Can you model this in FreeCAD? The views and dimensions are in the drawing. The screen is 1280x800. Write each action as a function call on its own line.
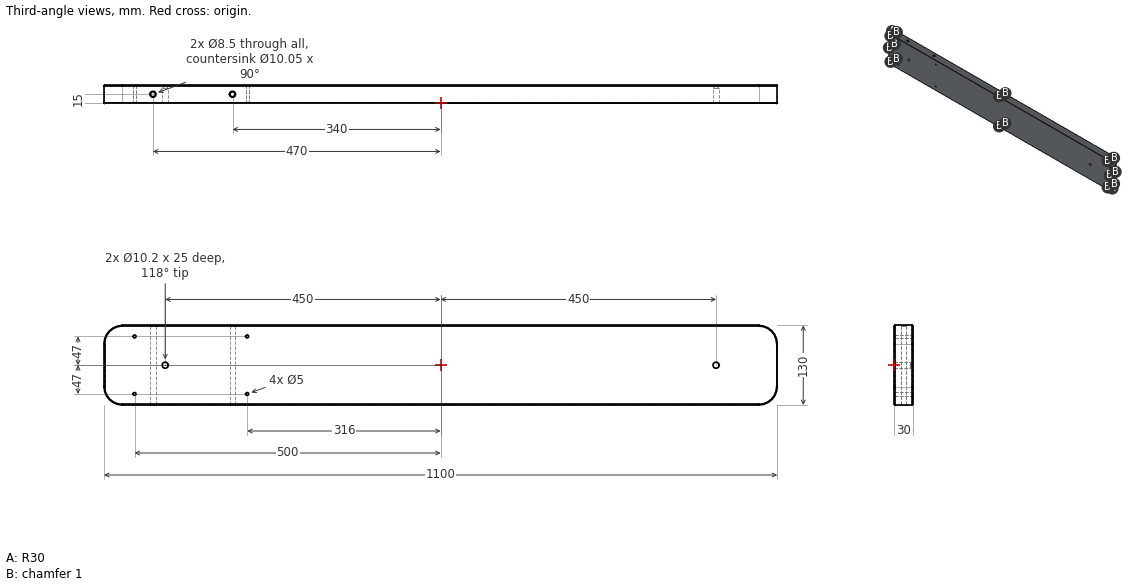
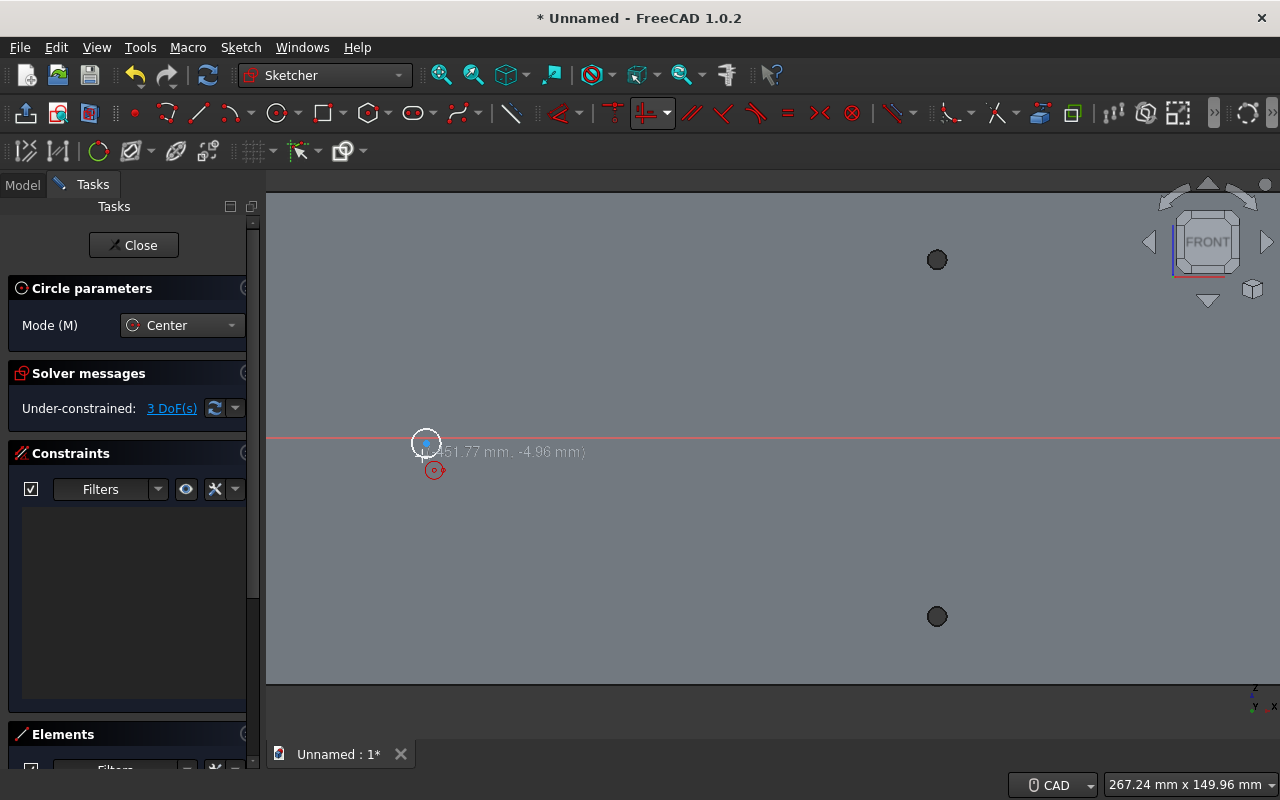
scroll(421, 458, down, 9)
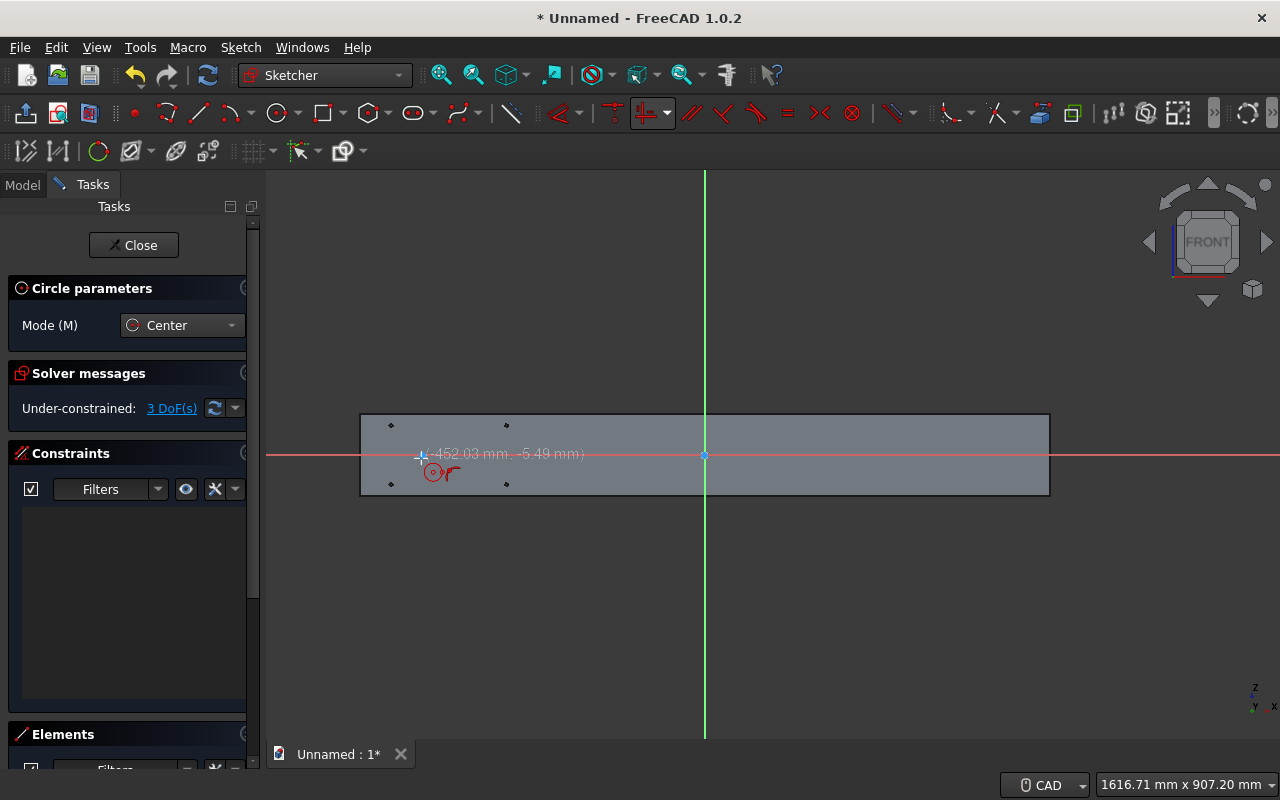
scroll(987, 455, up, 10)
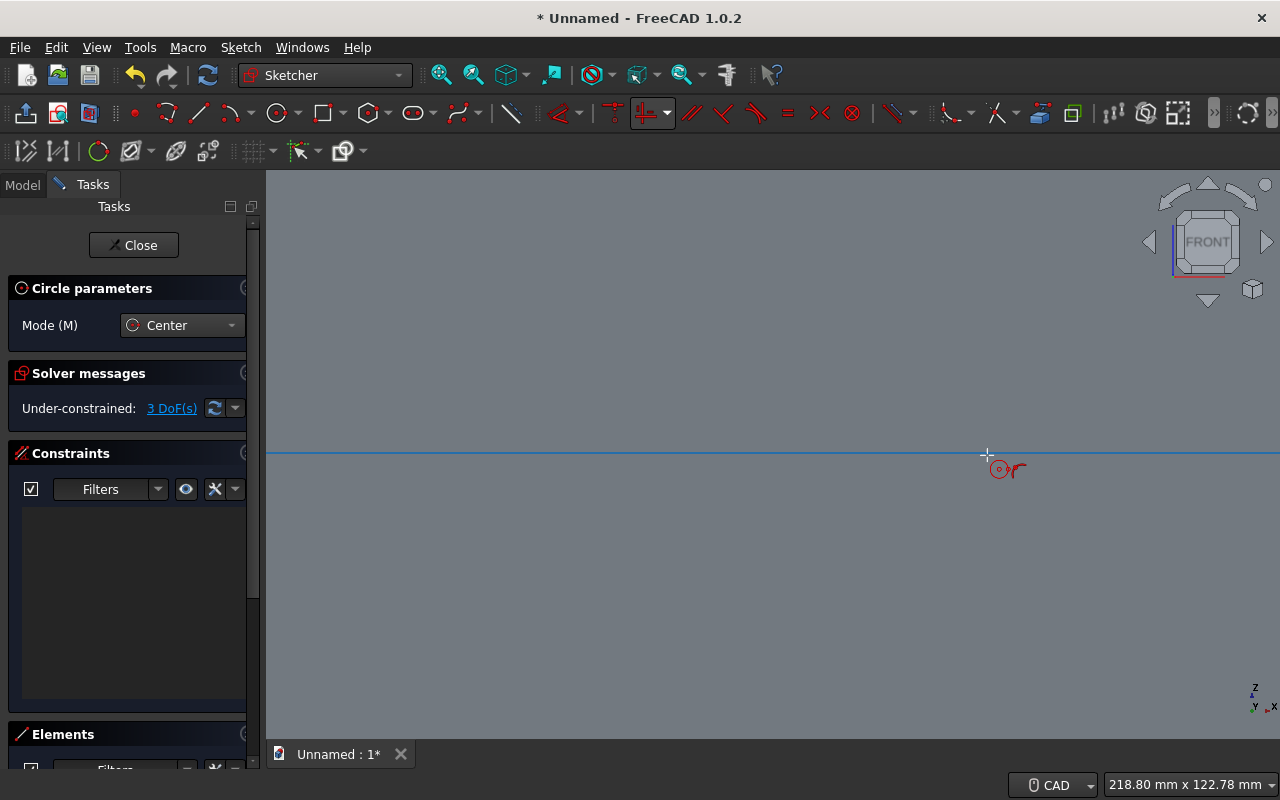
scroll(988, 455, down, 10)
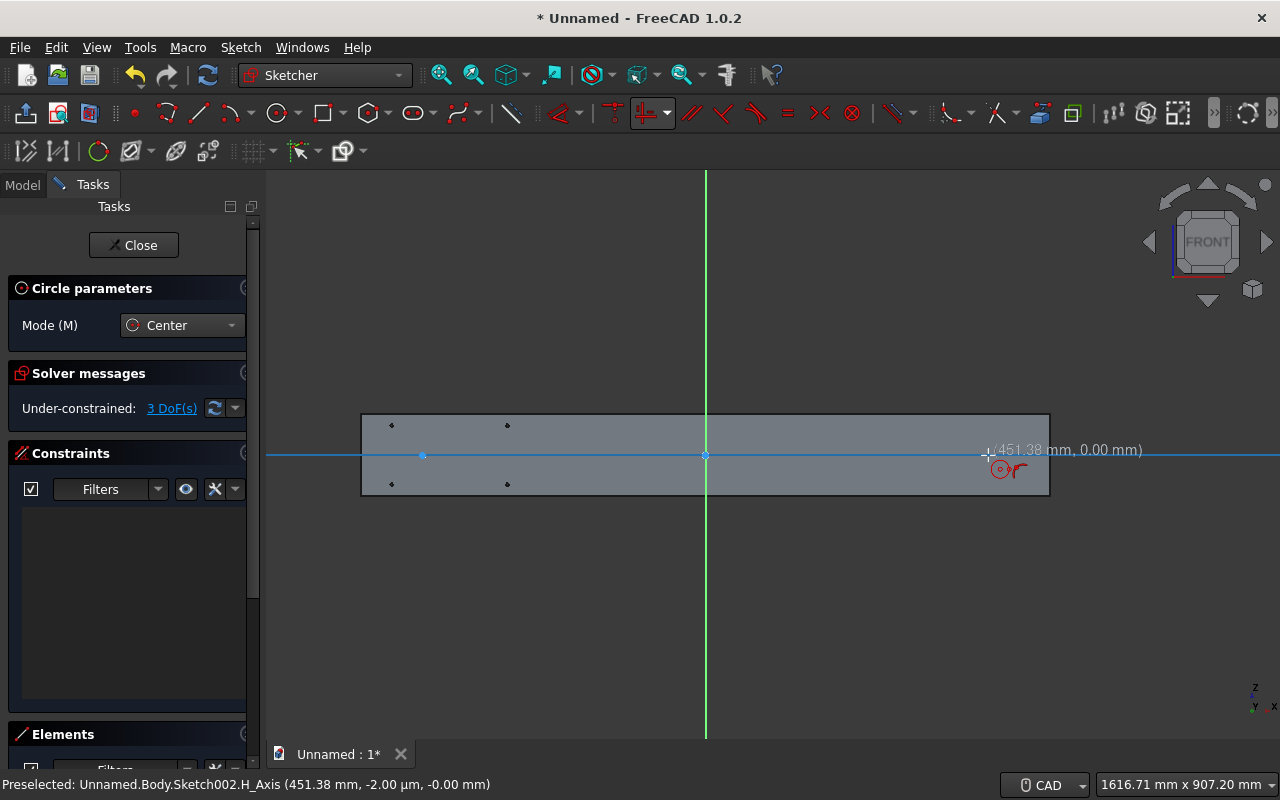
click(988, 455)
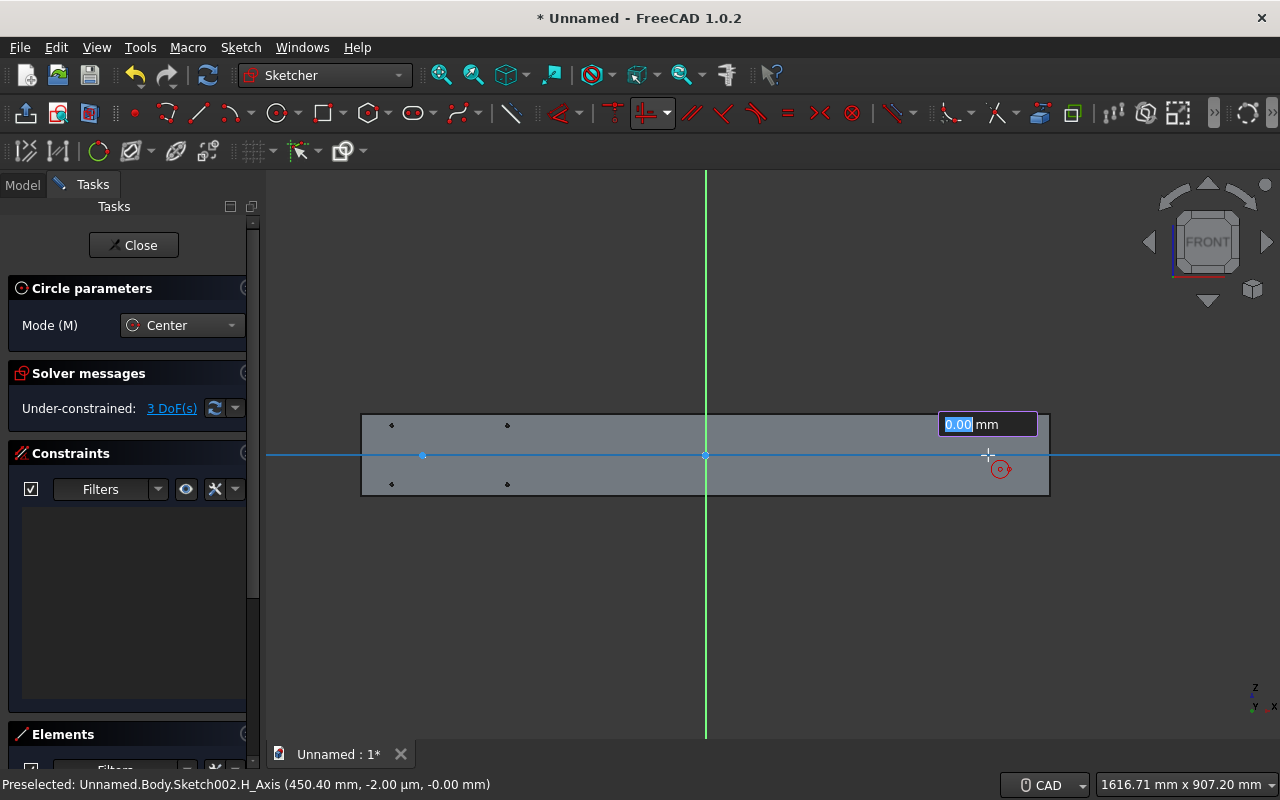
scroll(987, 458, up, 9)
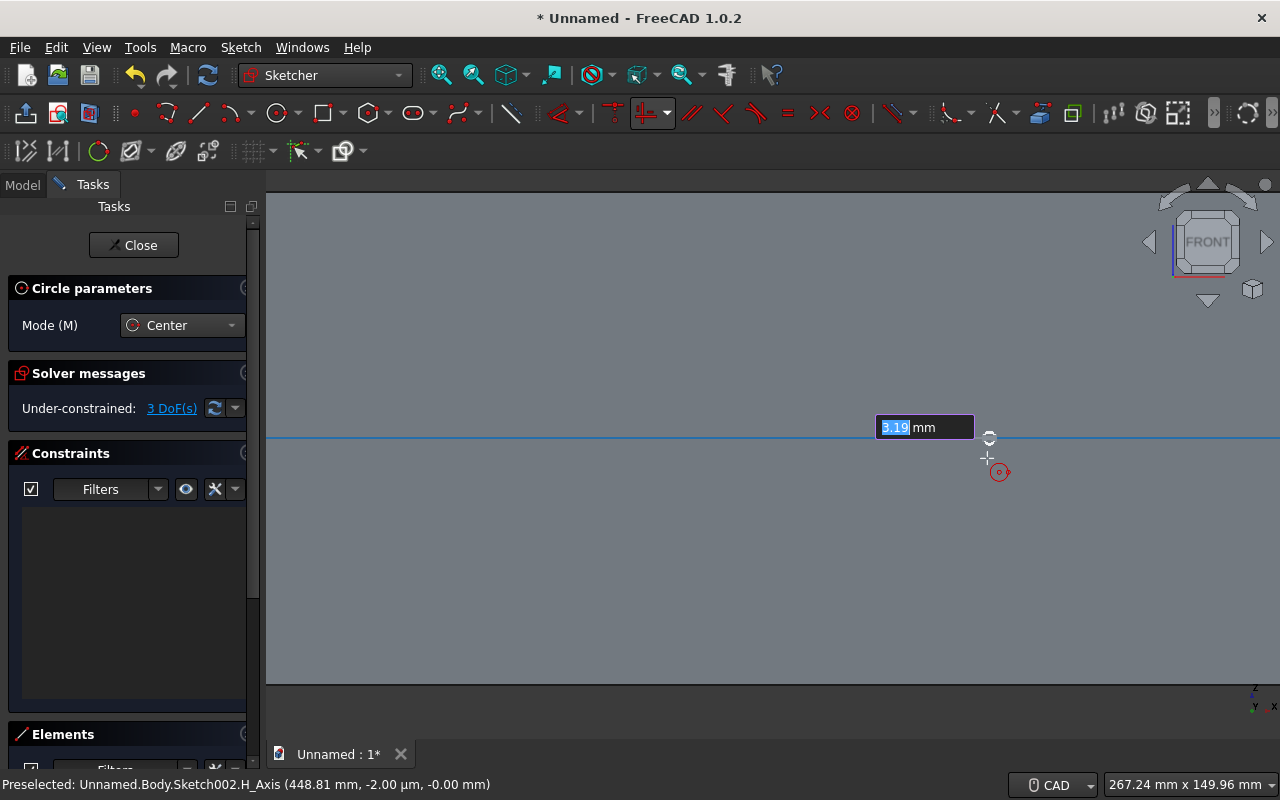
click(981, 456)
key(Escape)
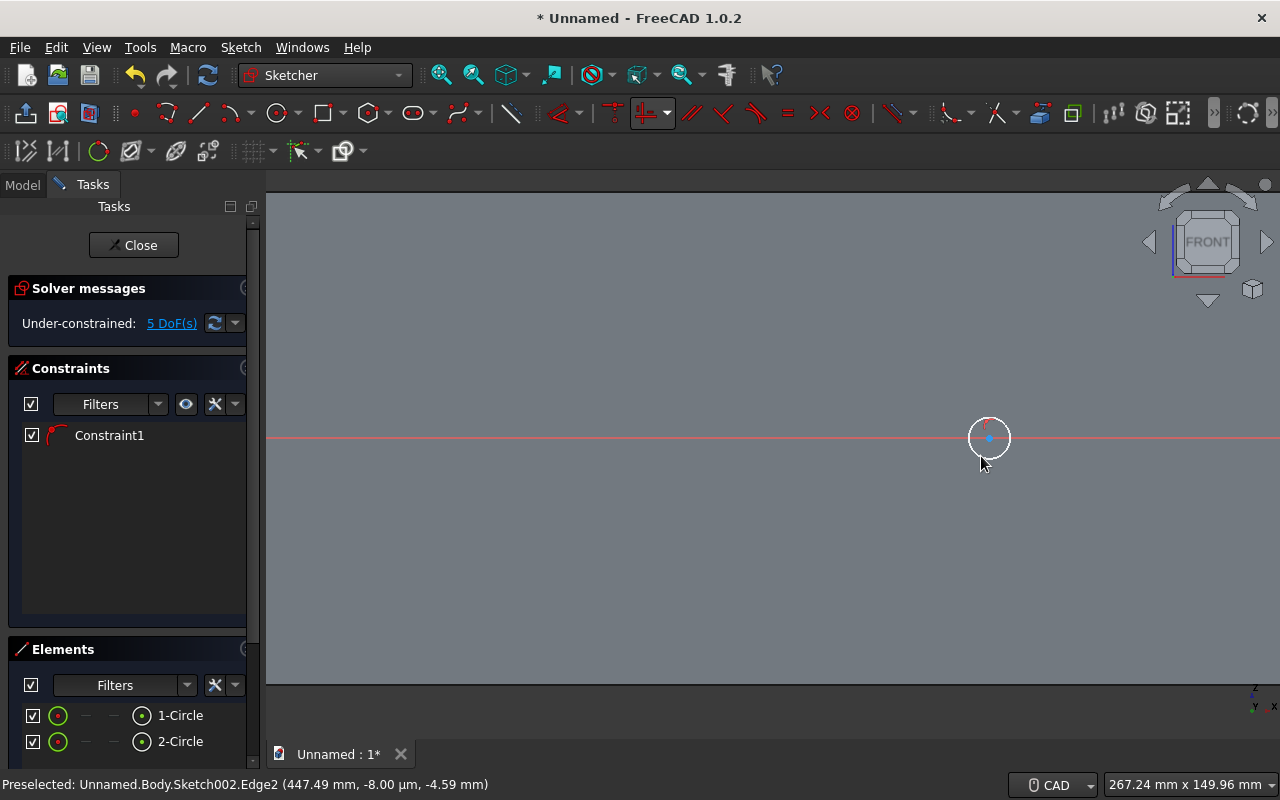
scroll(987, 458, down, 9)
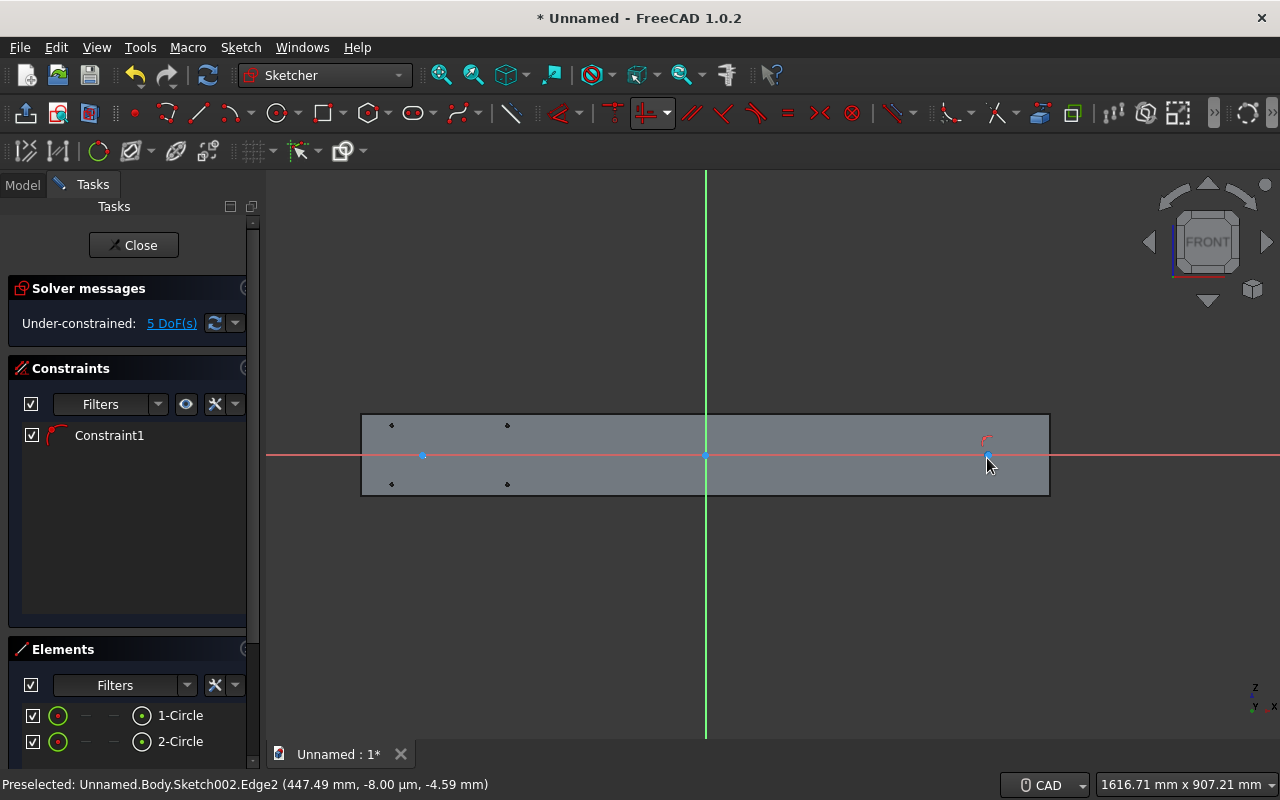
scroll(421, 458, up, 9)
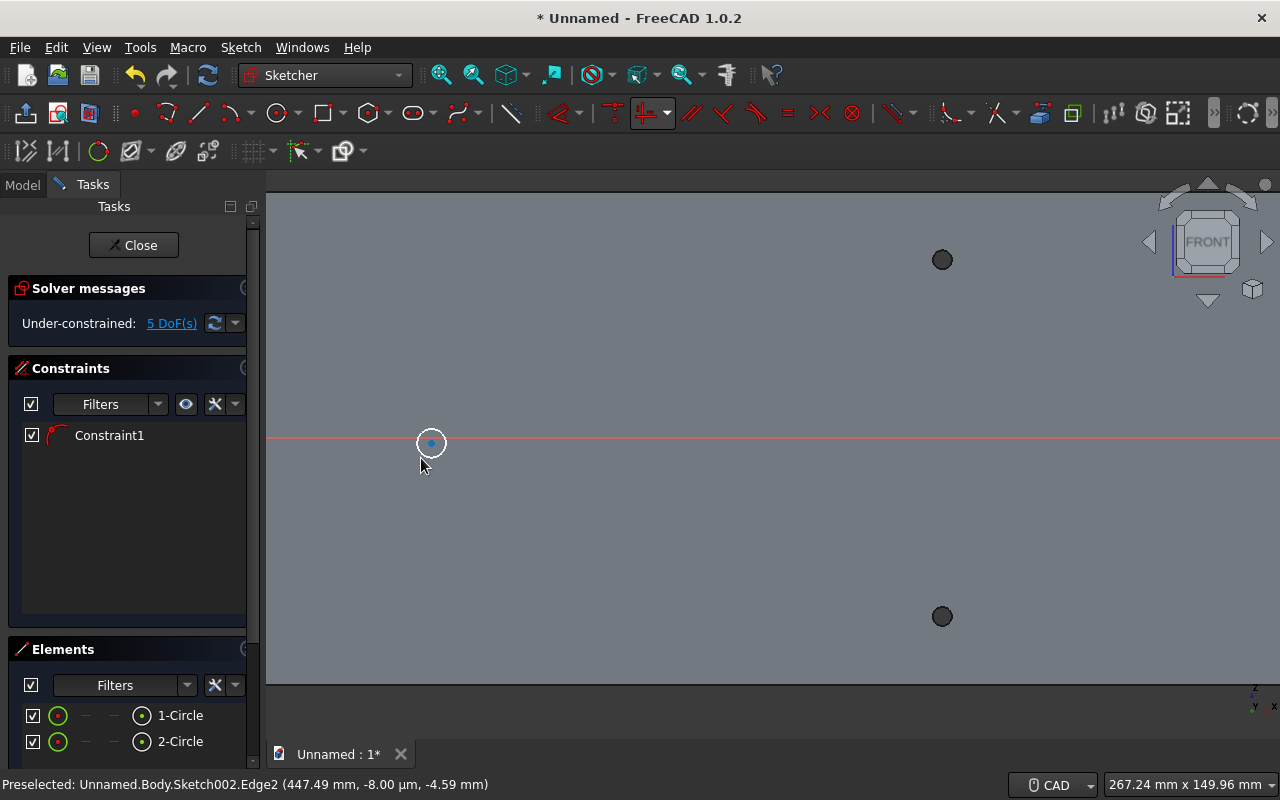
click(421, 453)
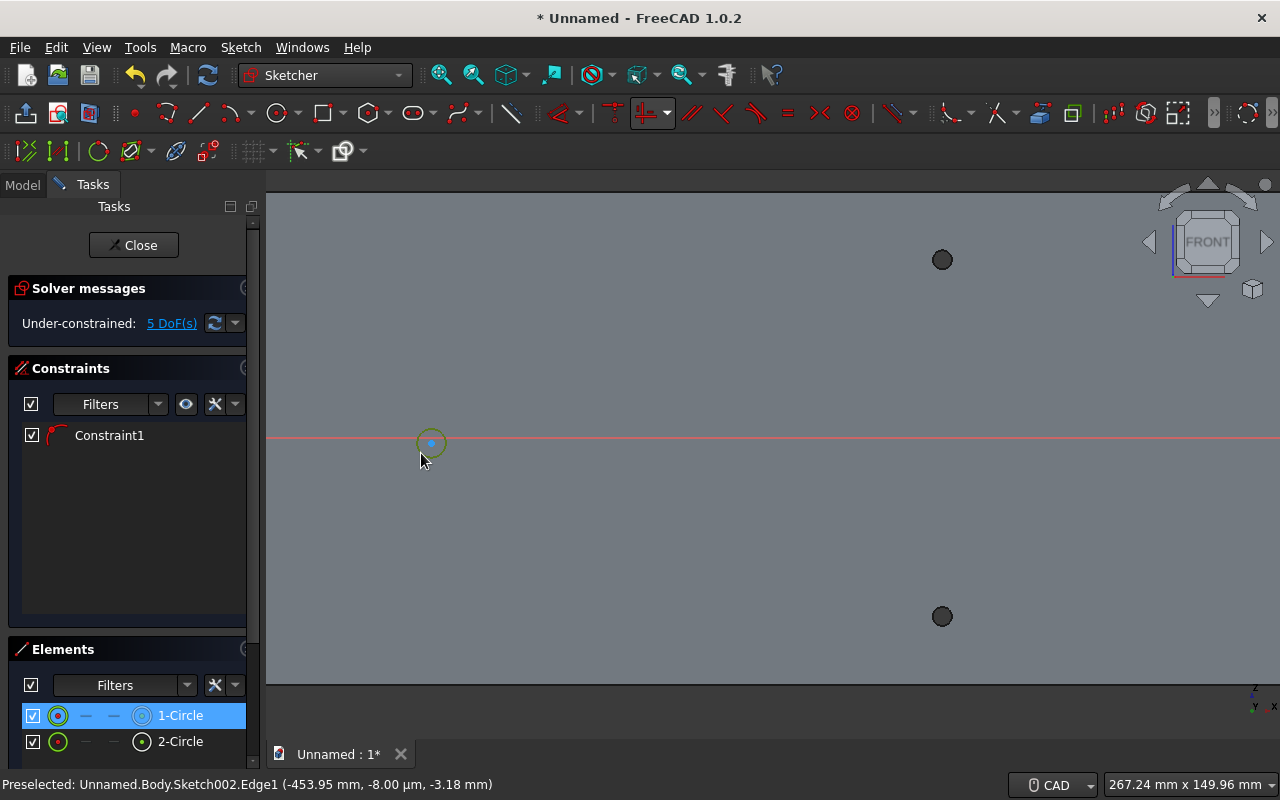
scroll(420, 458, down, 9)